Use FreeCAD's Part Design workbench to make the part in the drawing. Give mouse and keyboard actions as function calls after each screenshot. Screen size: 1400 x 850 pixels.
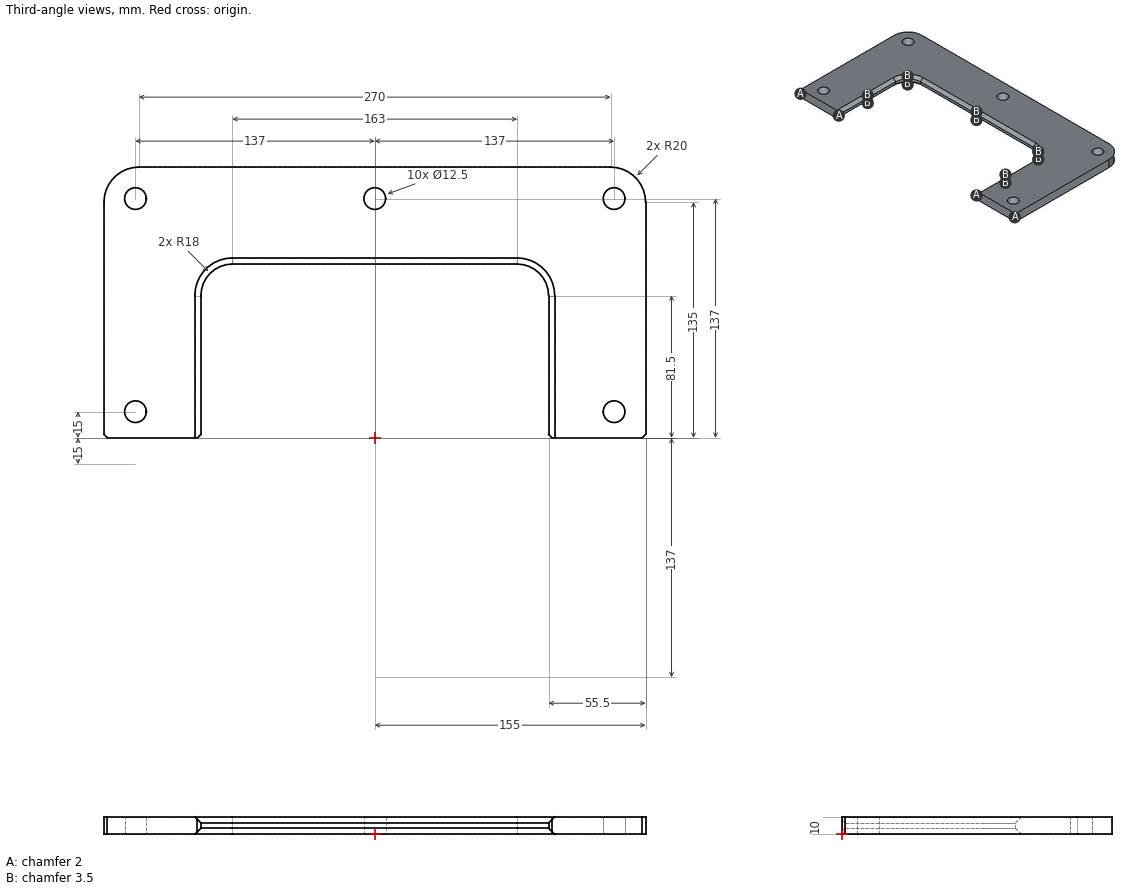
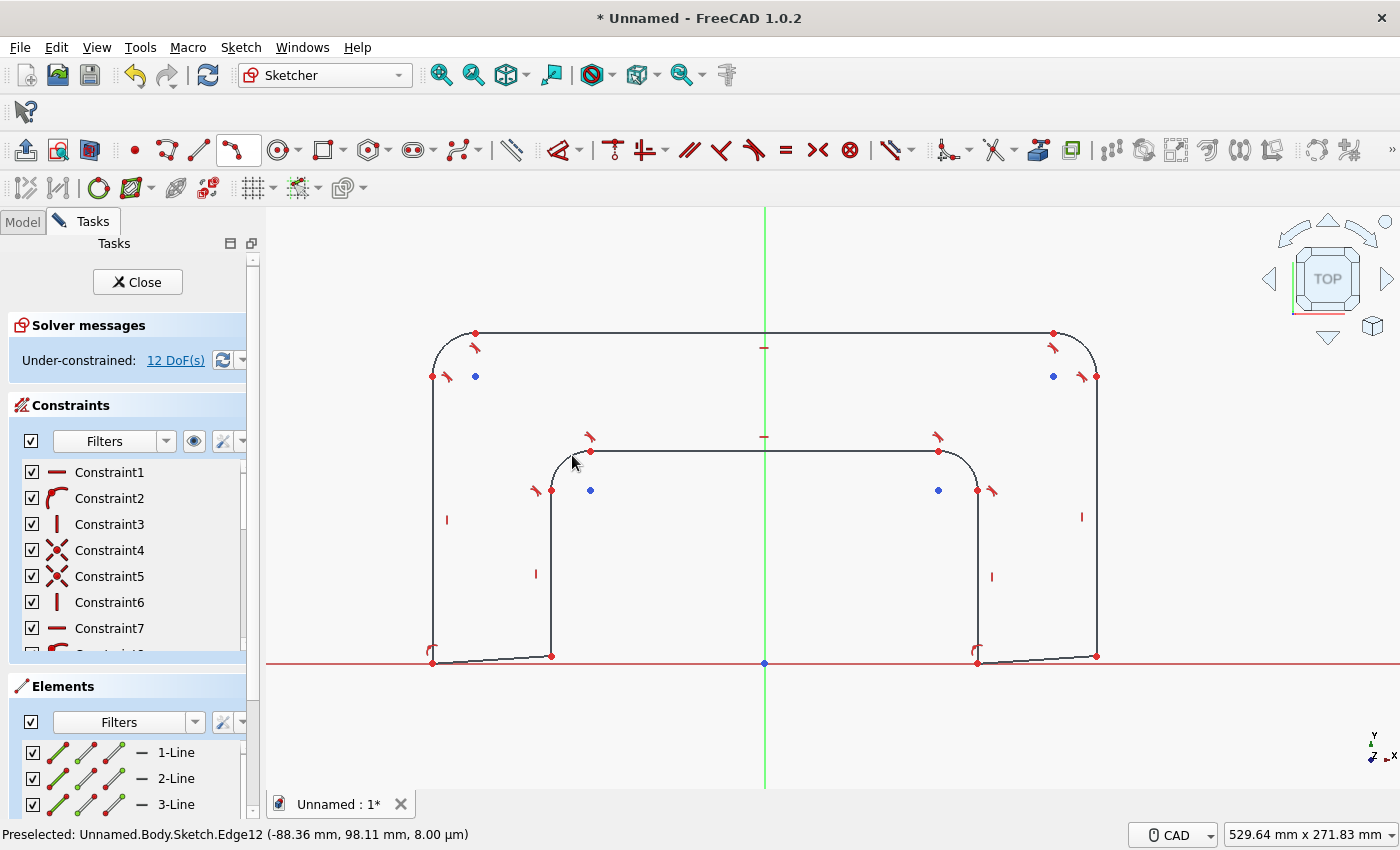
click(1013, 662)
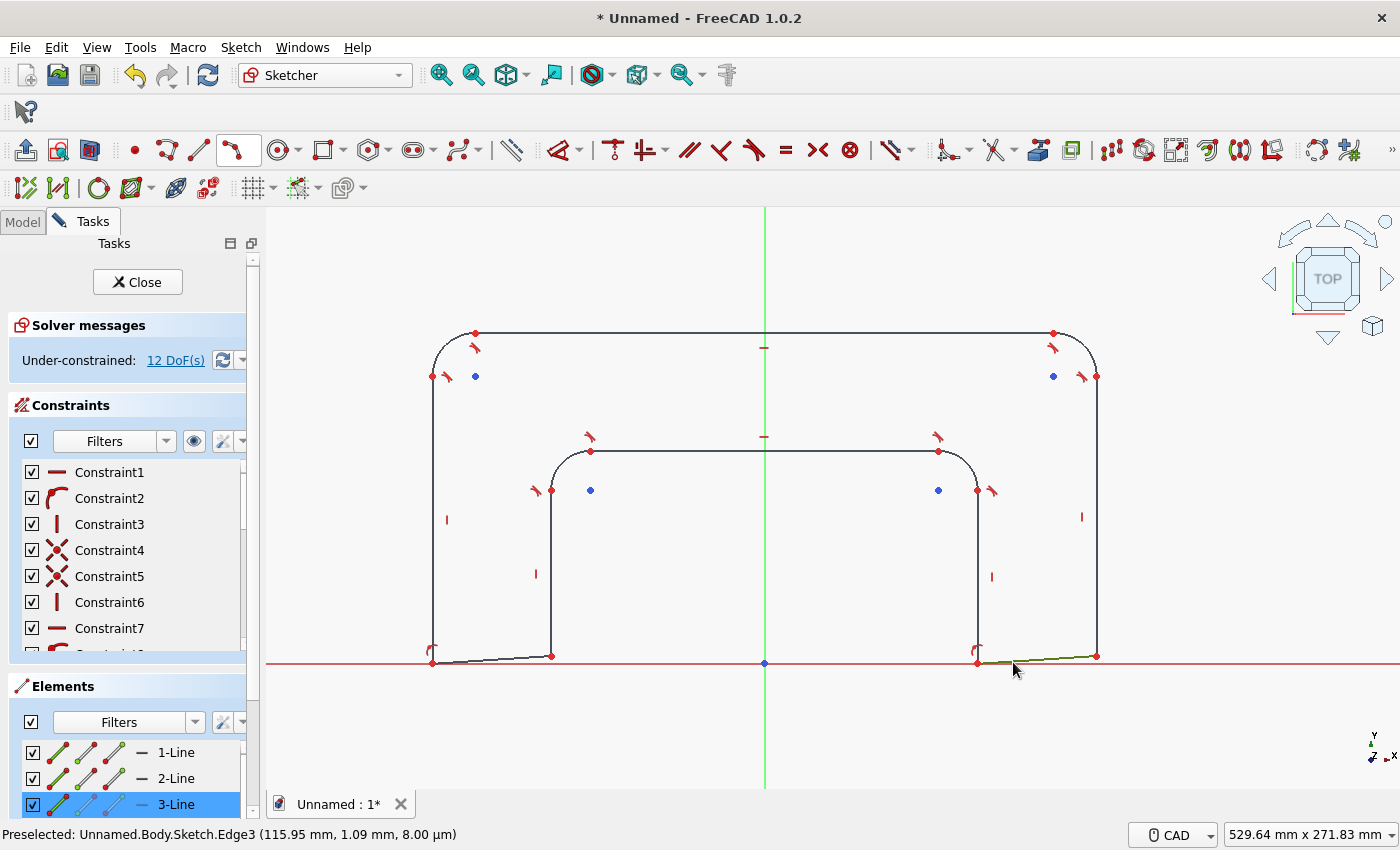
key(h)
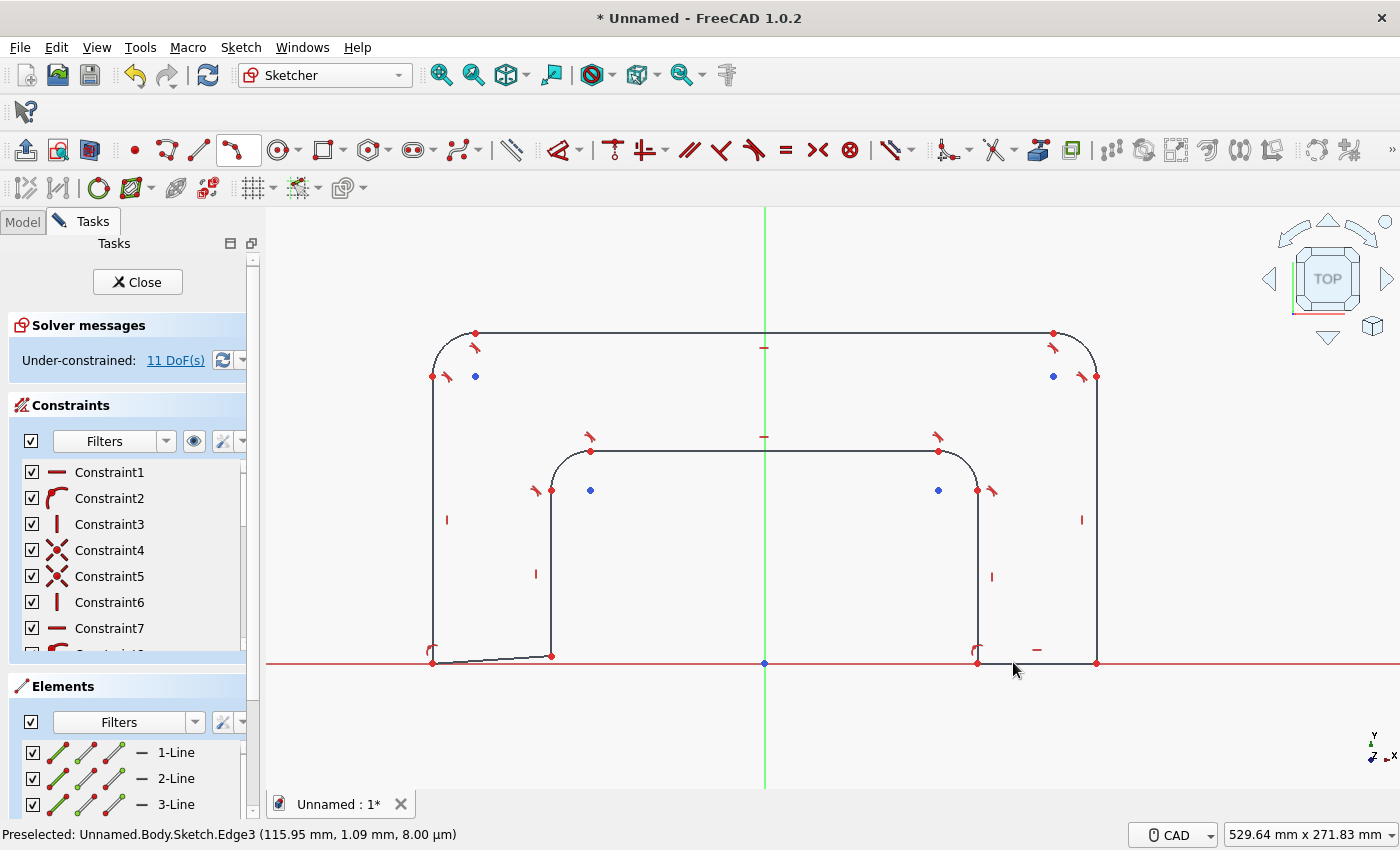
click(468, 662)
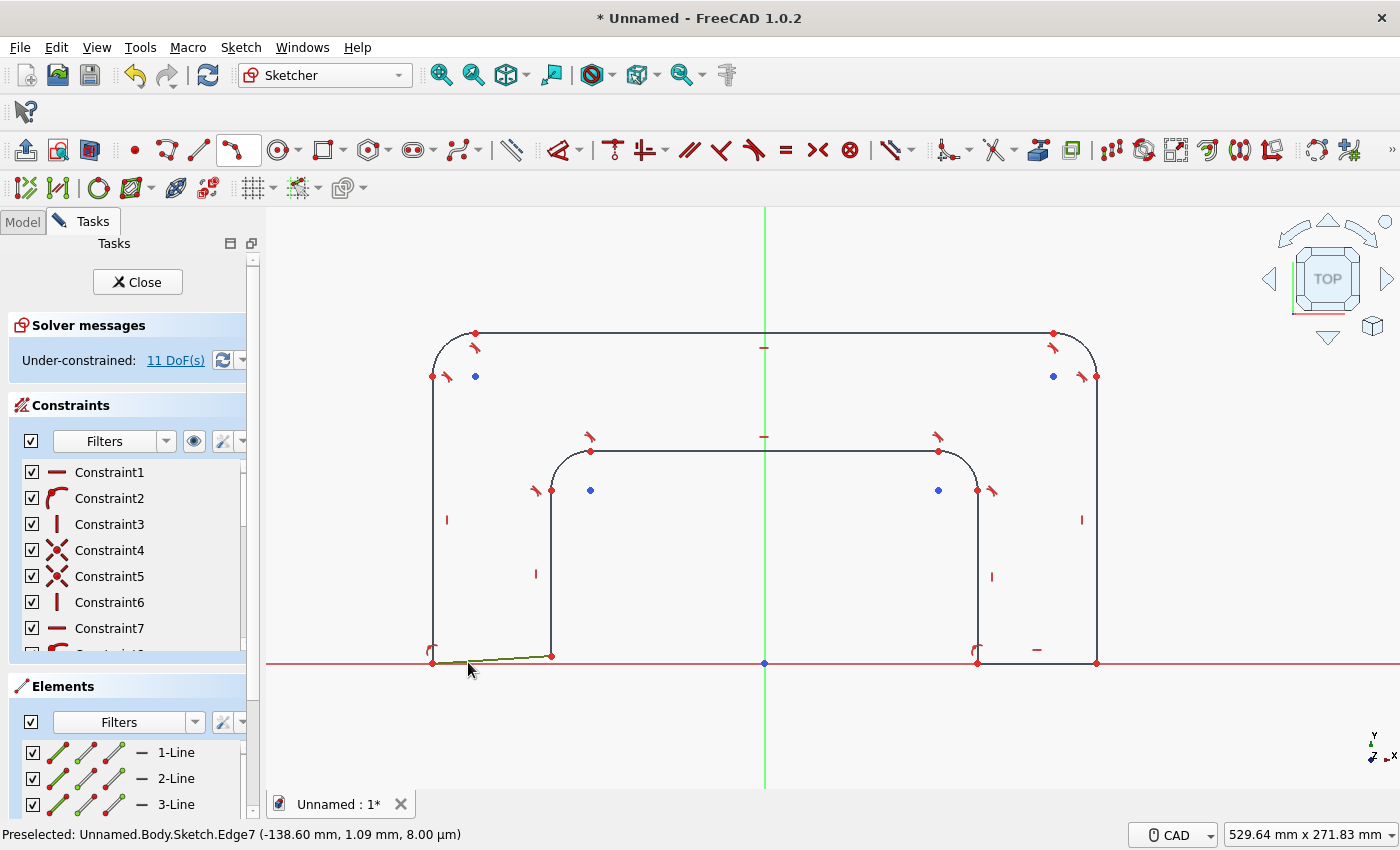
click(668, 150)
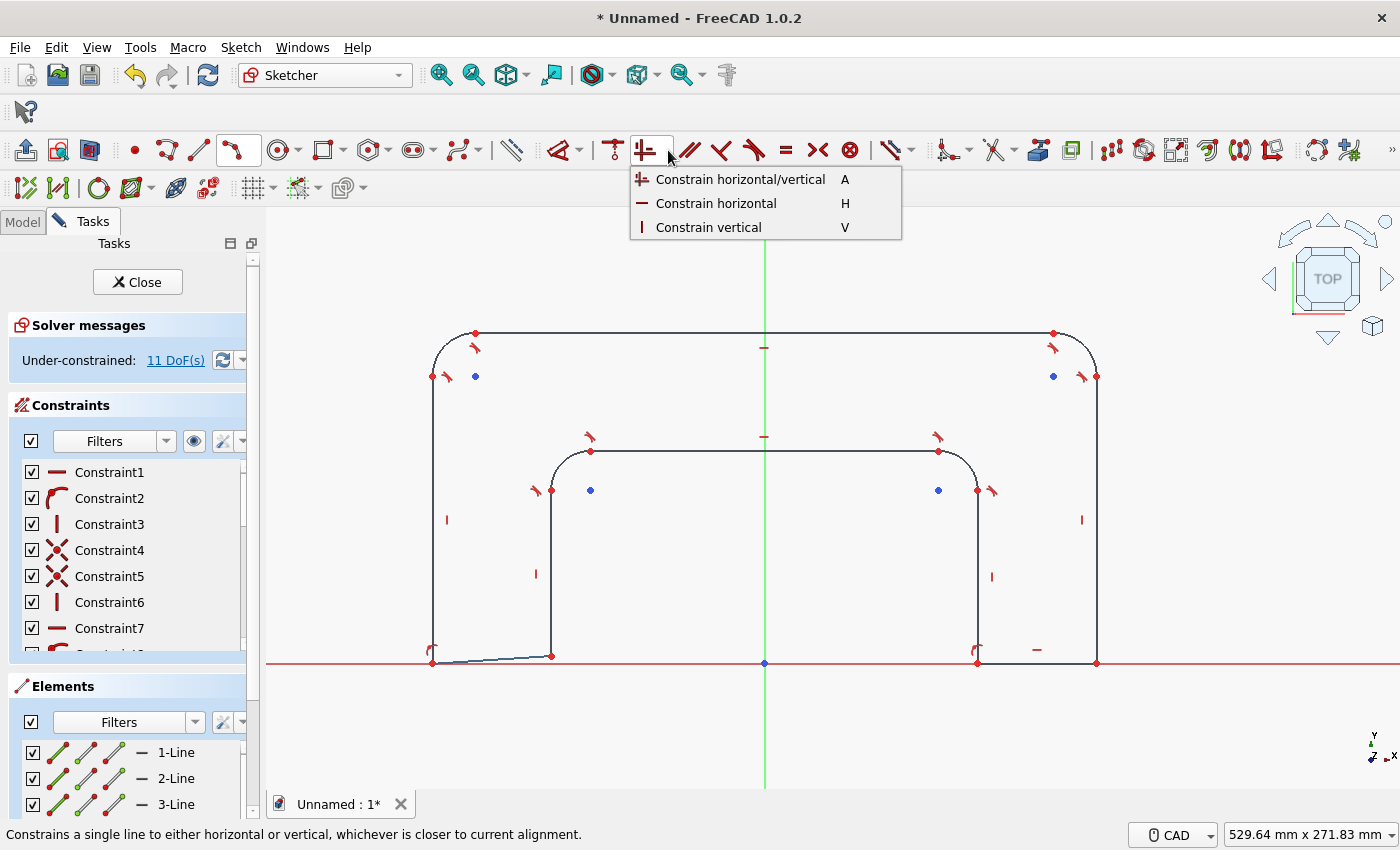
click(766, 203)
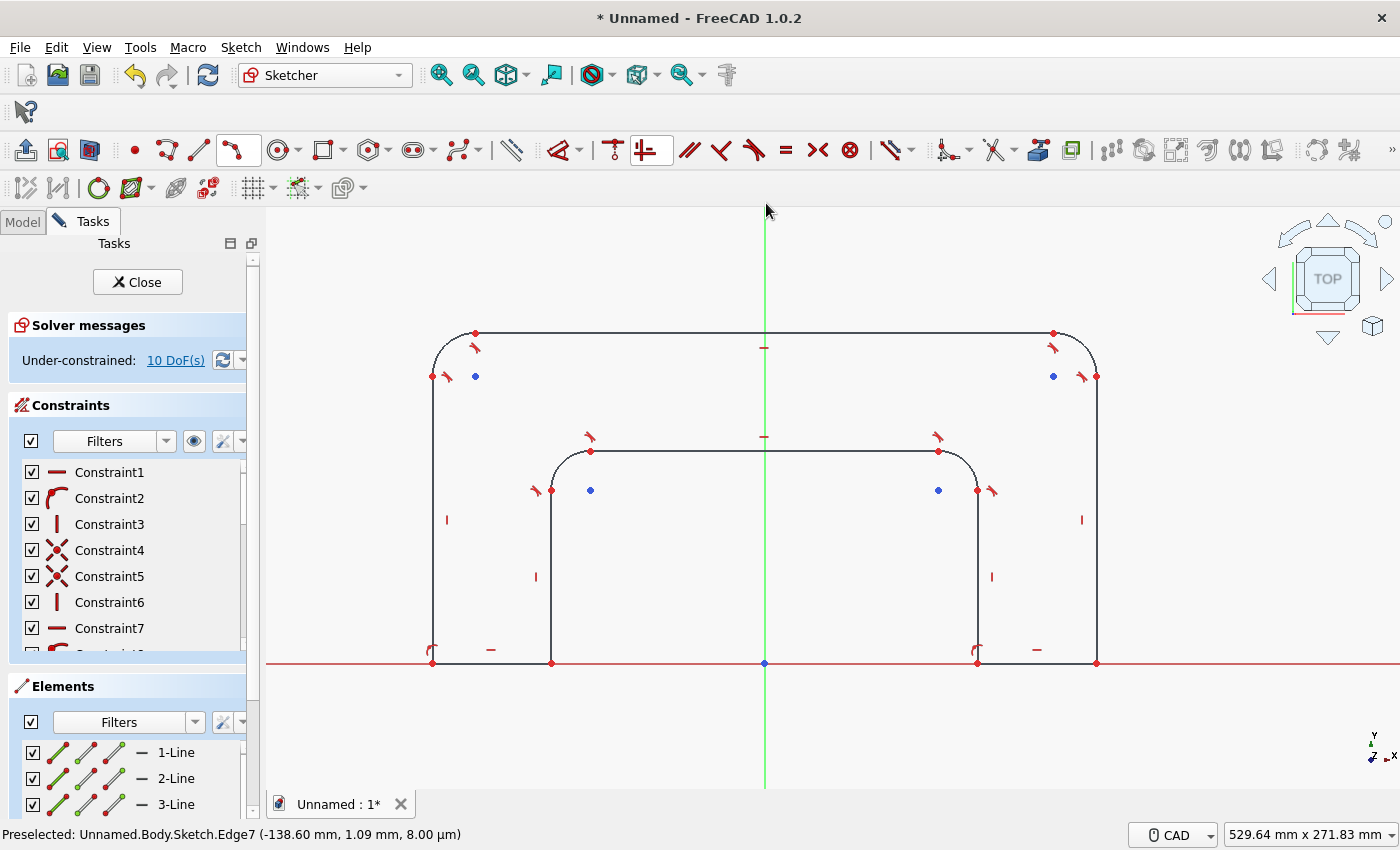
click(1092, 356)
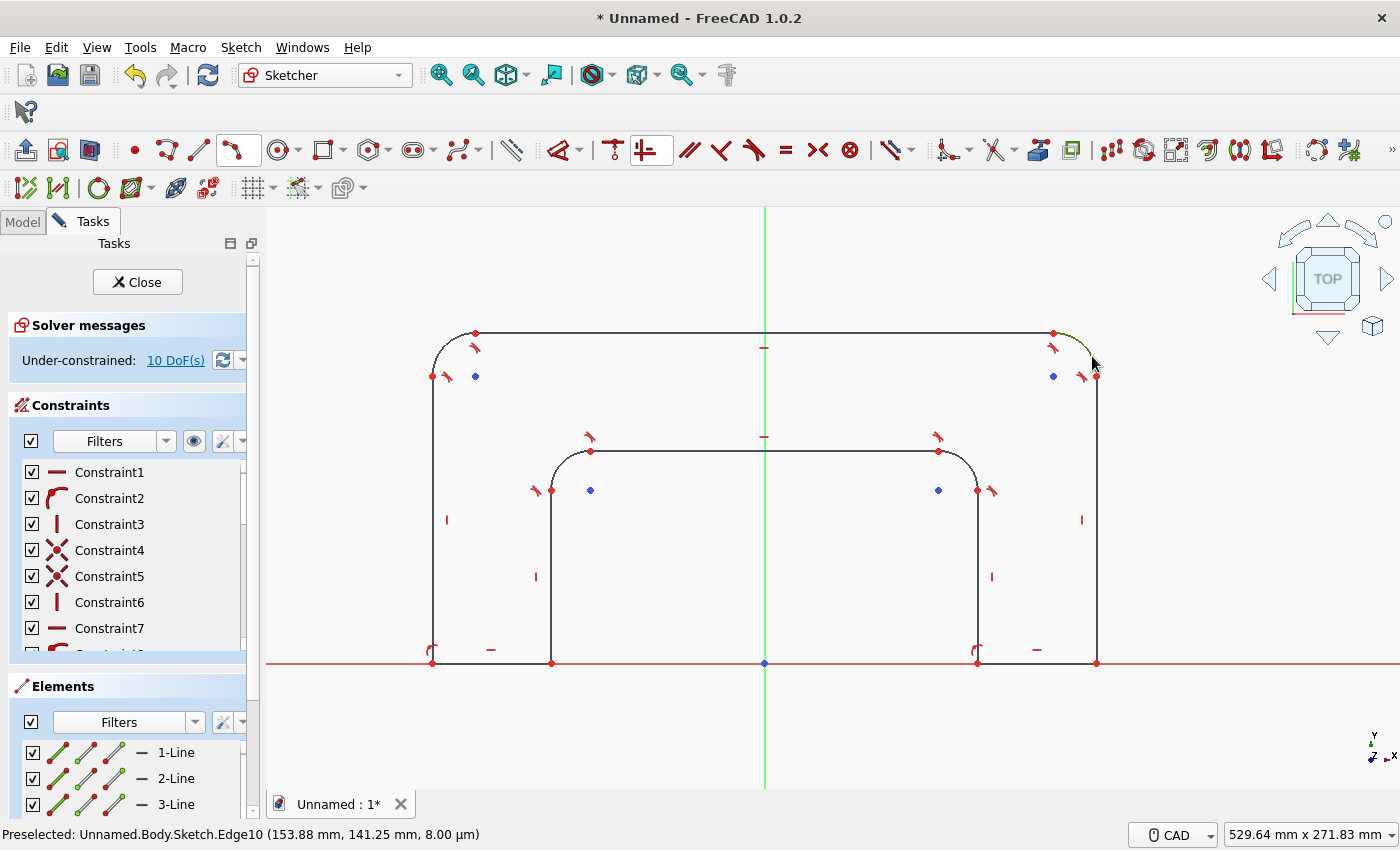
click(456, 338)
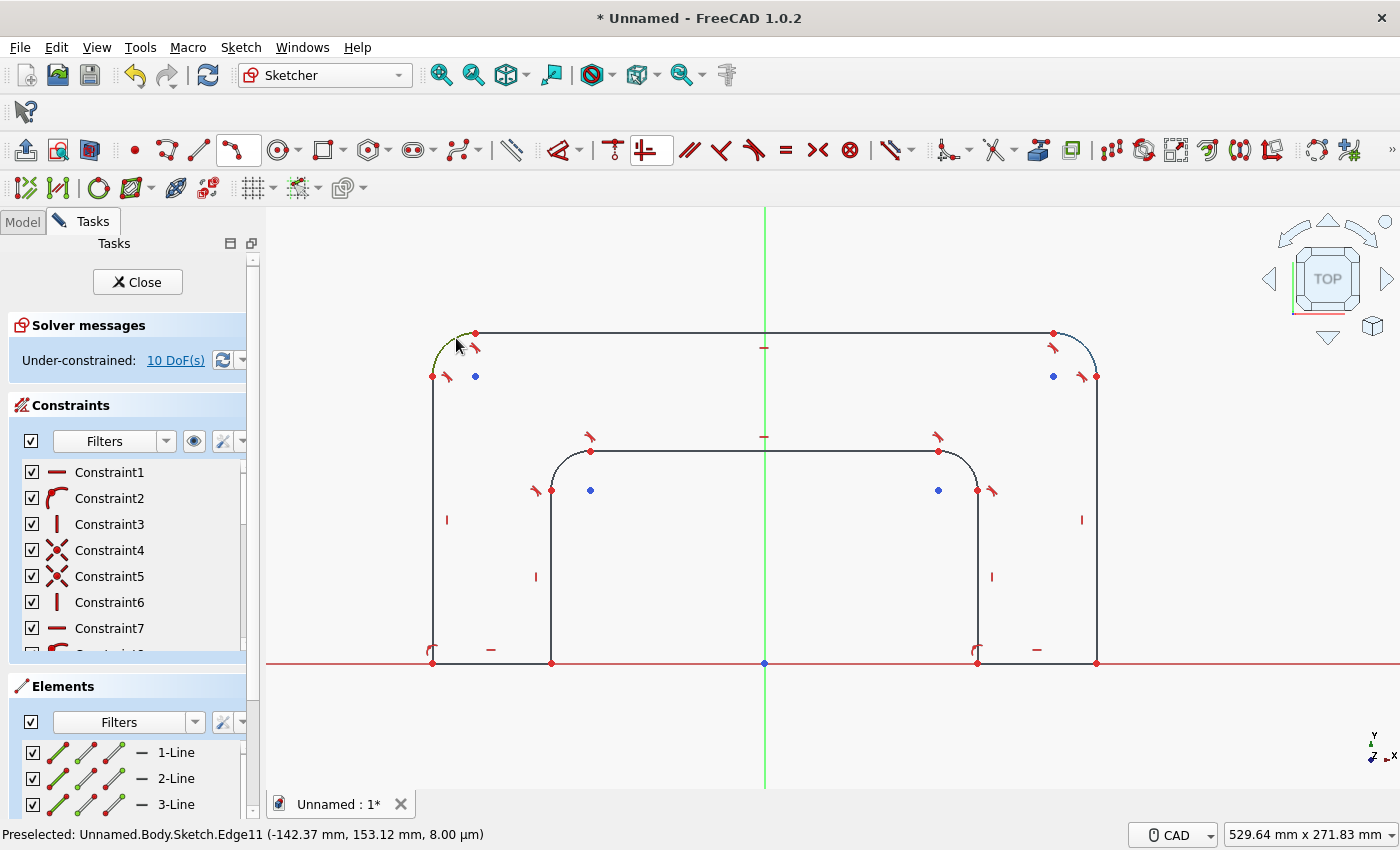
click(786, 150)